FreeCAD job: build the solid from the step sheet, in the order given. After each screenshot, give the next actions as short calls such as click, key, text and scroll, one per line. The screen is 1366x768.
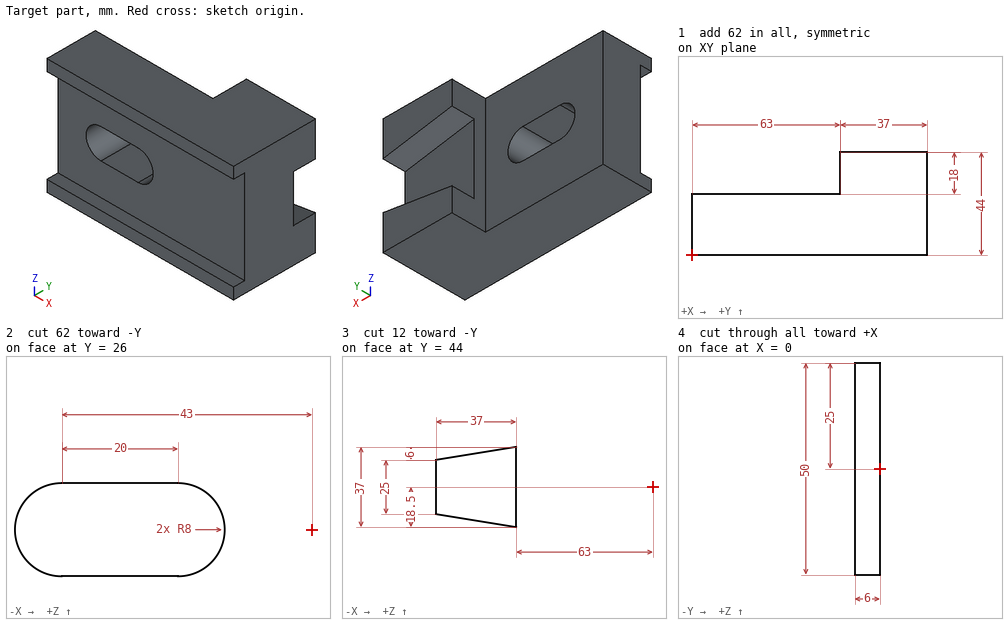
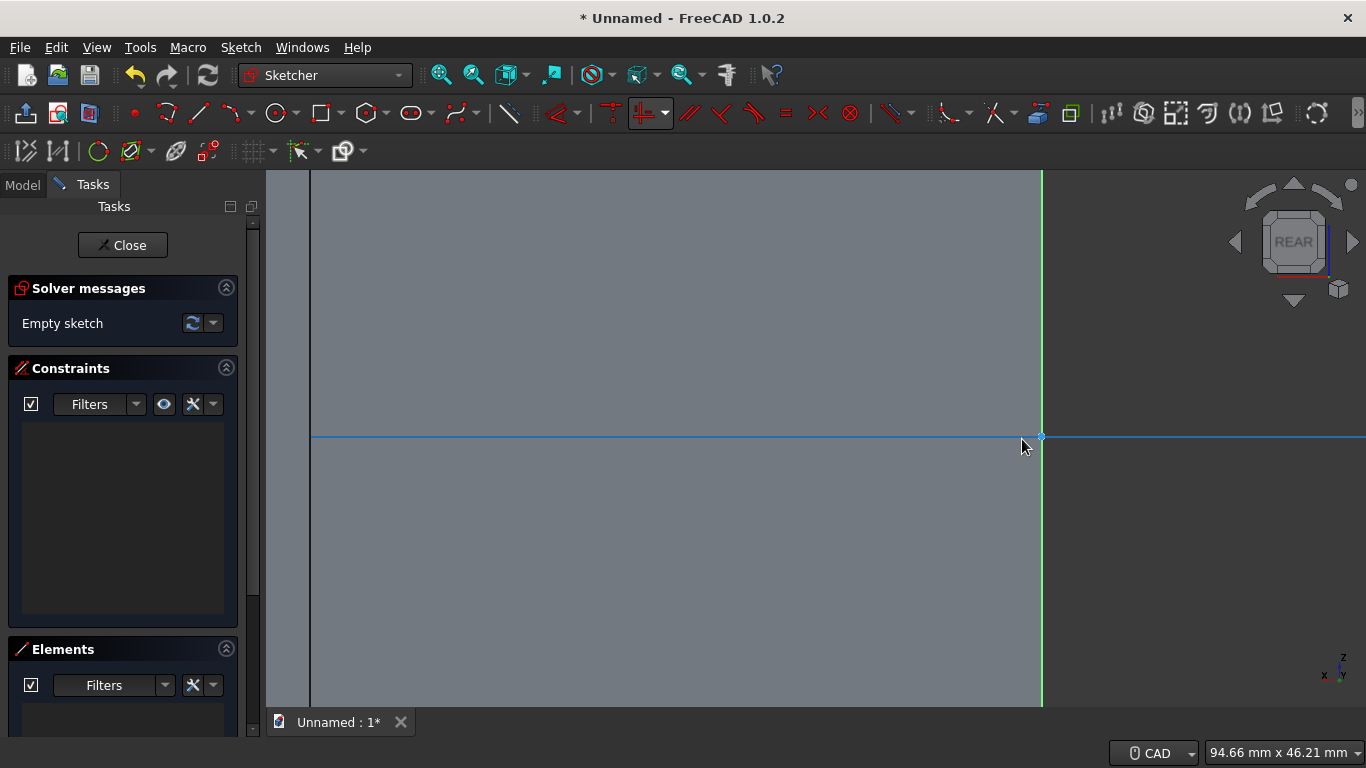
click(412, 114)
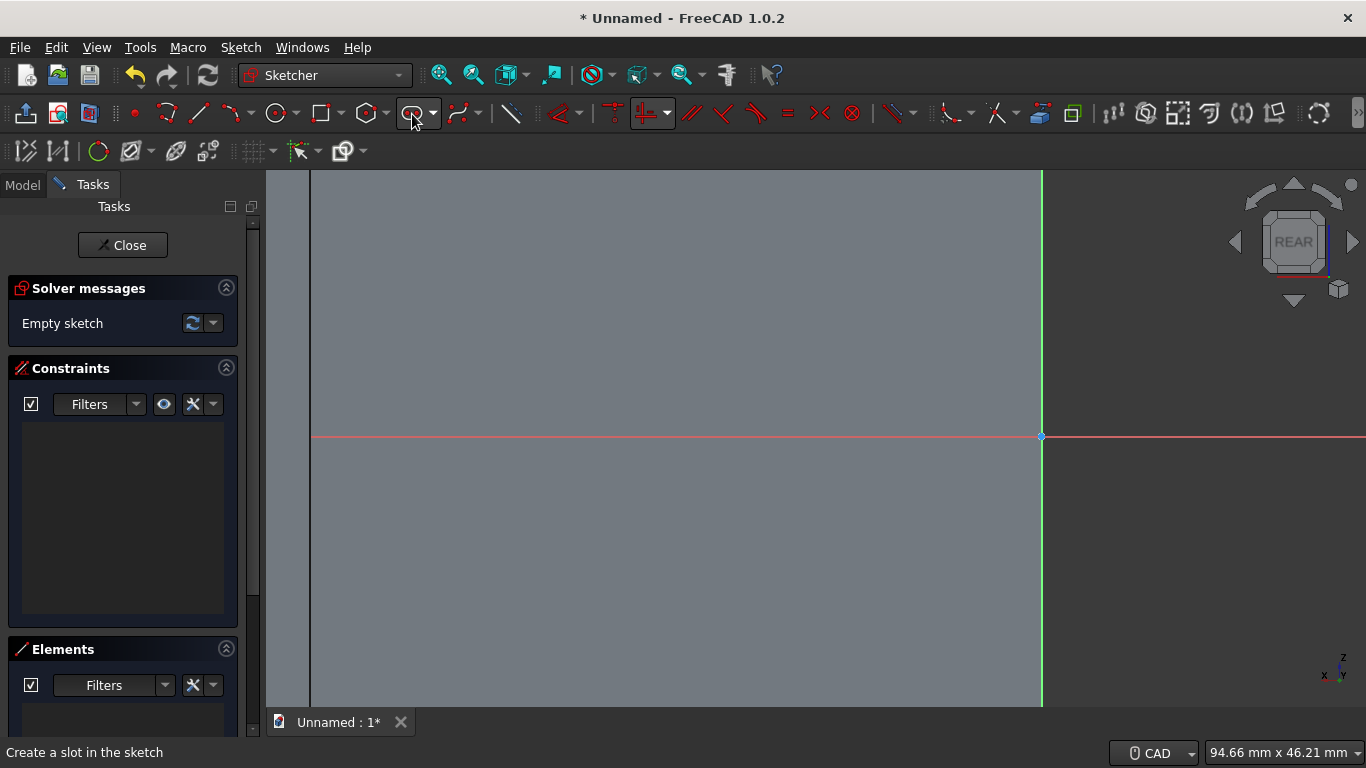
click(542, 437)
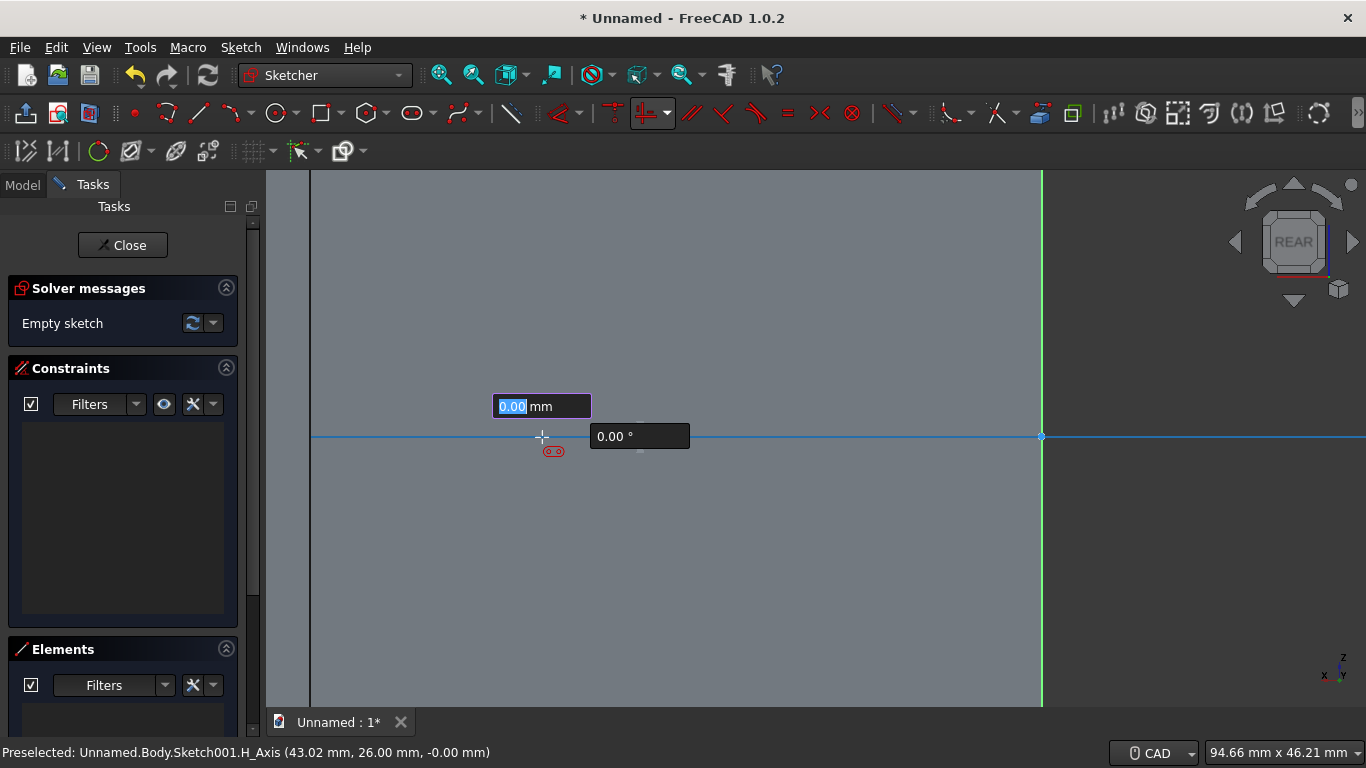
click(775, 428)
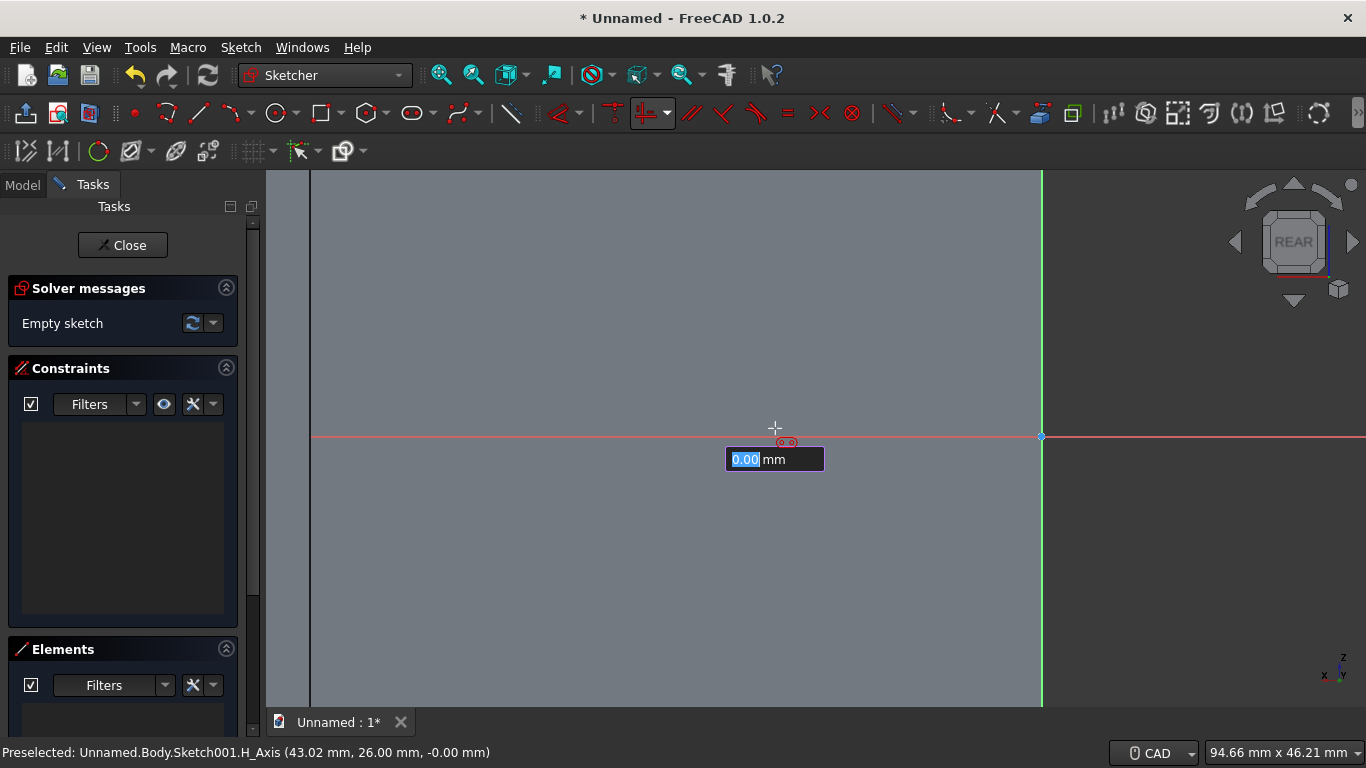
click(658, 530)
key(Escape)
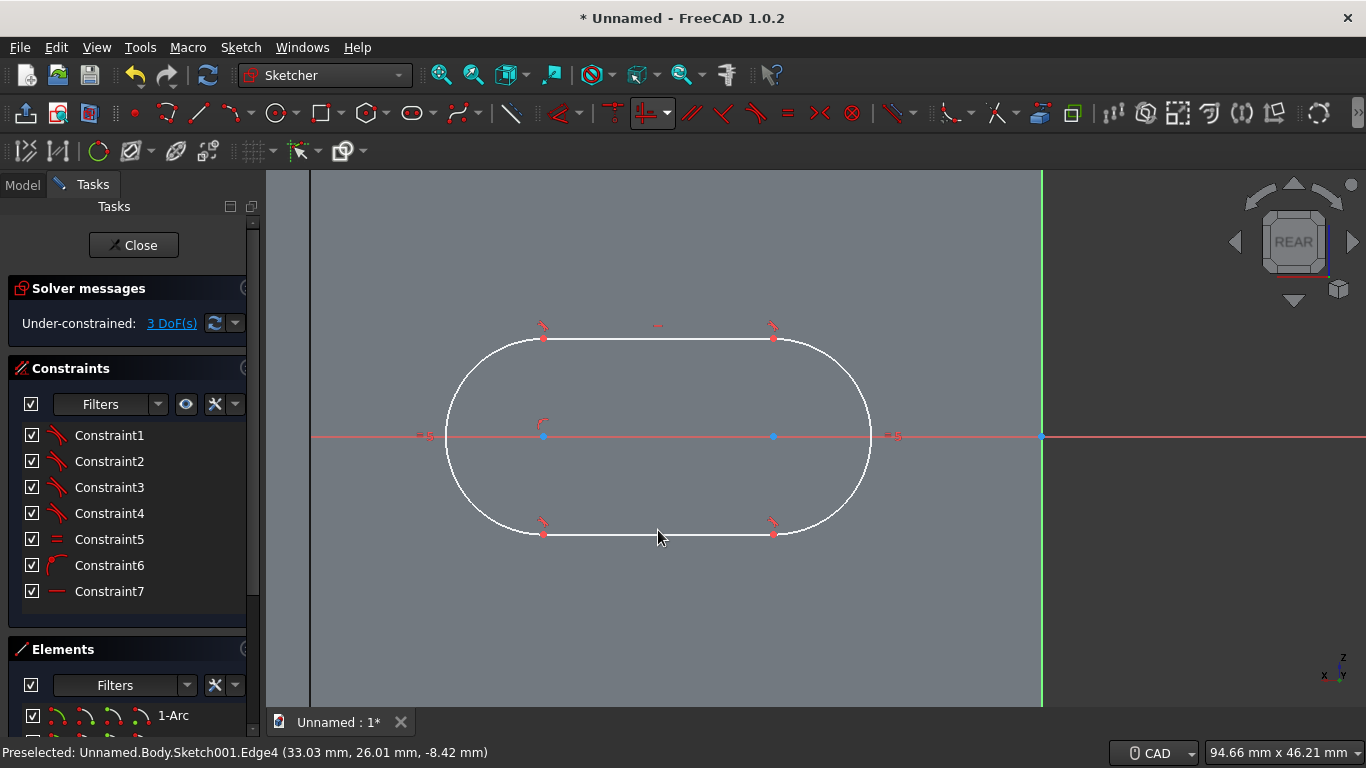
click(558, 114)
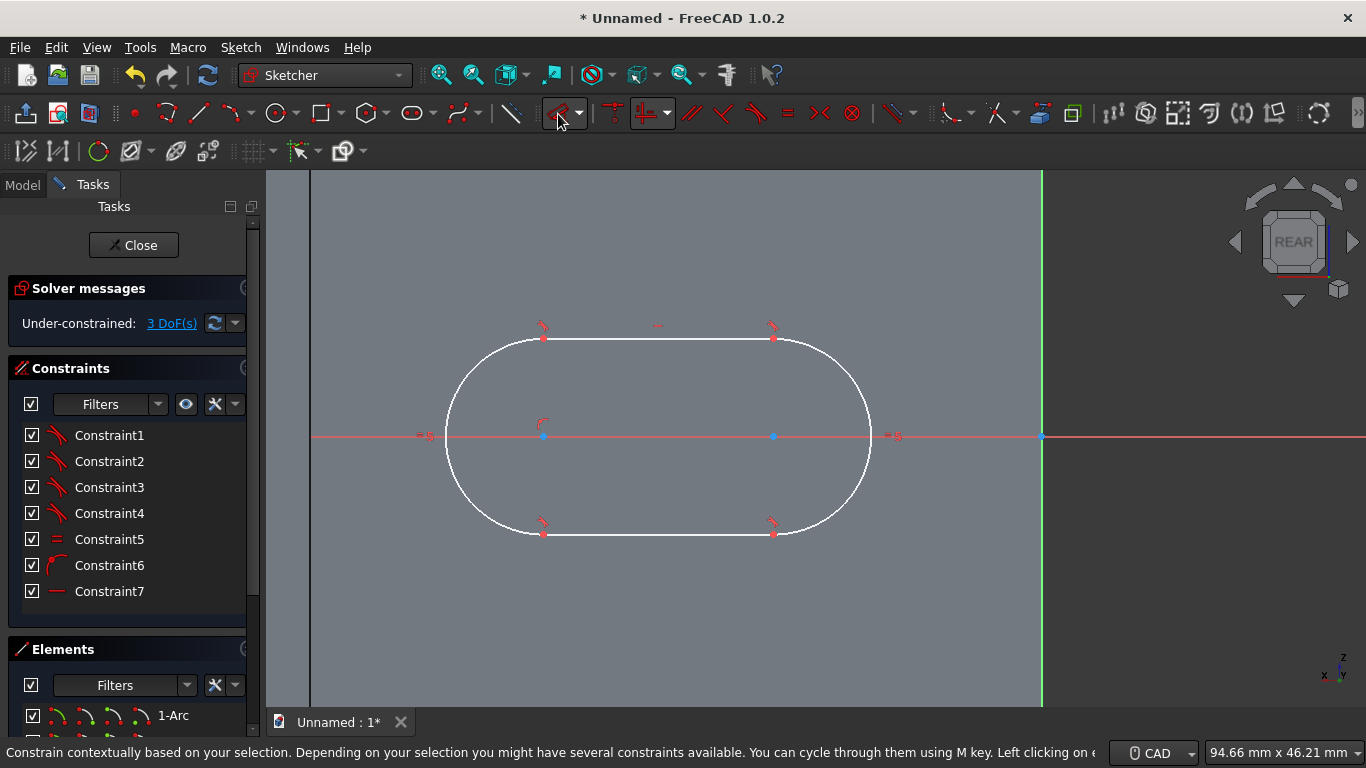
click(465, 379)
click(439, 360)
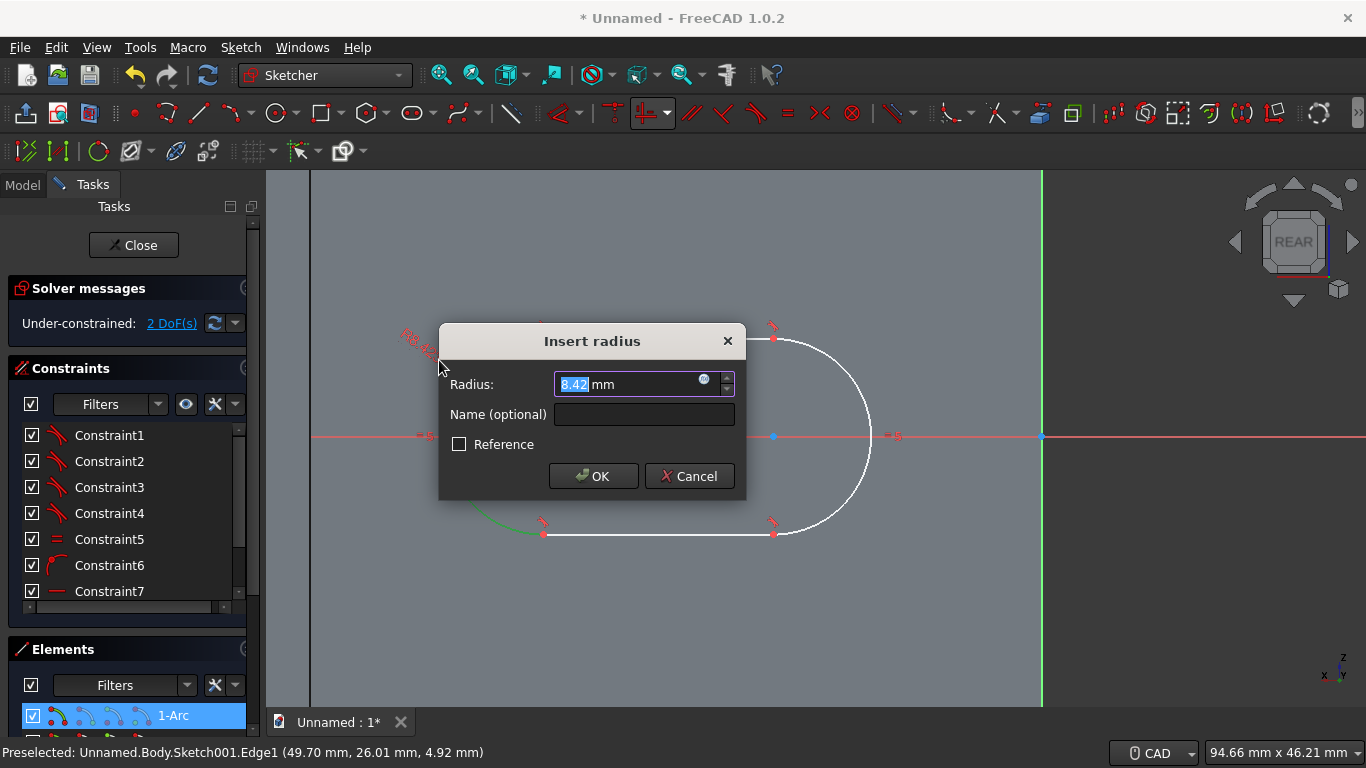
text(8)
key(Return)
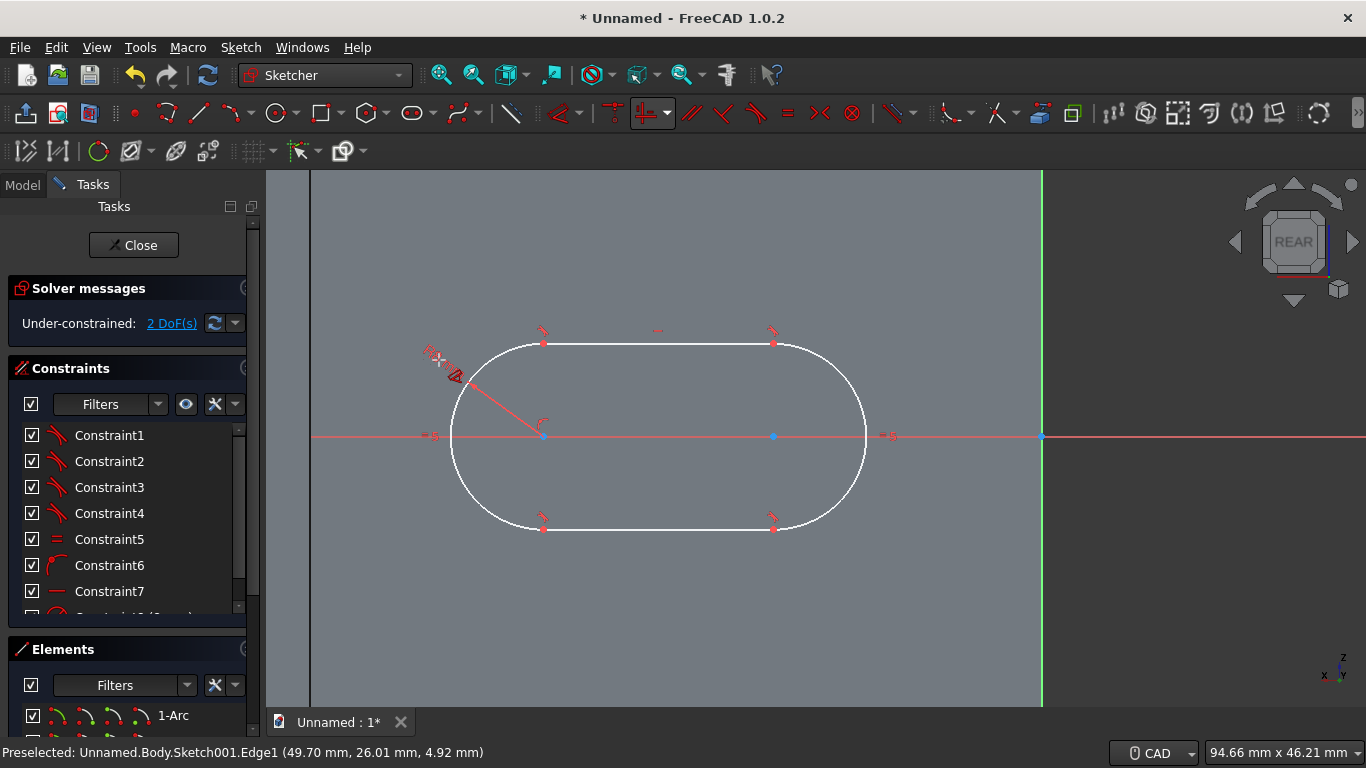
click(613, 344)
click(658, 310)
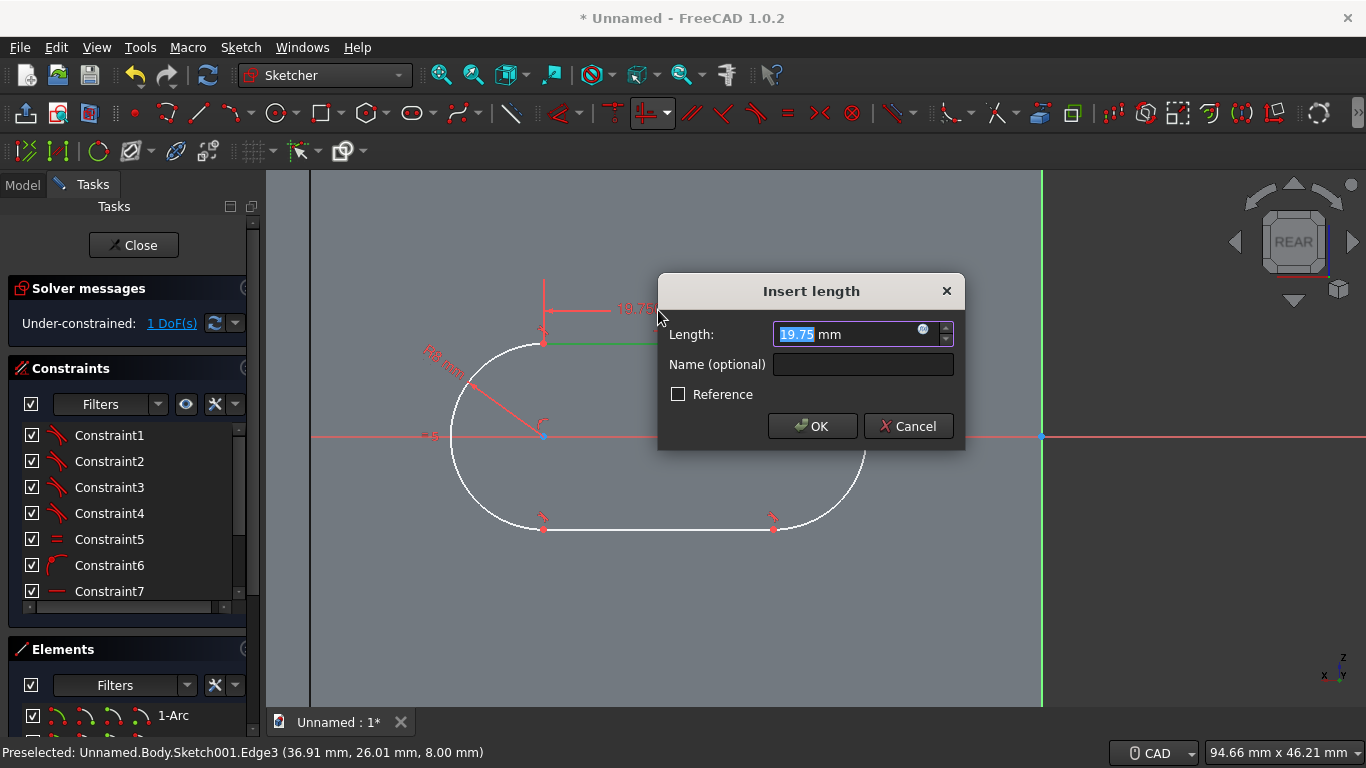
text(20)
key(Return)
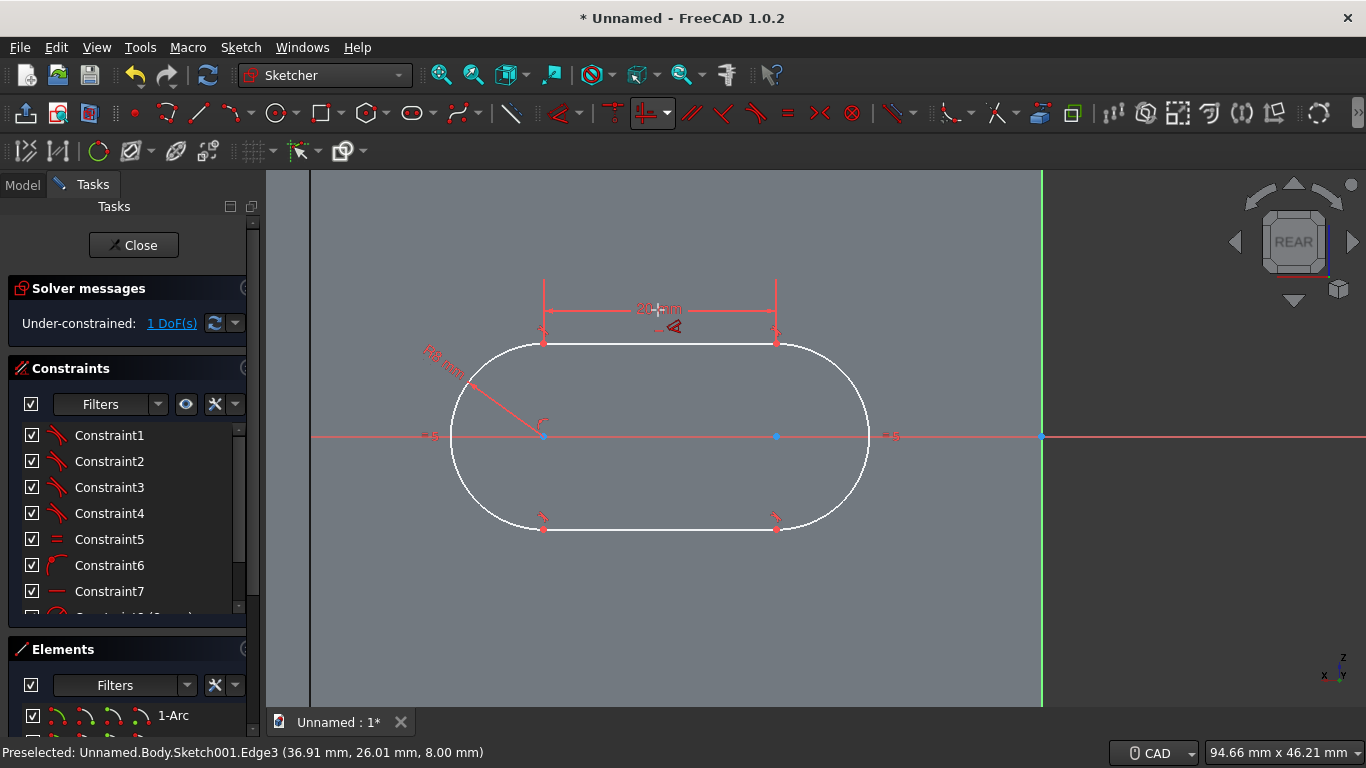
click(544, 344)
click(793, 310)